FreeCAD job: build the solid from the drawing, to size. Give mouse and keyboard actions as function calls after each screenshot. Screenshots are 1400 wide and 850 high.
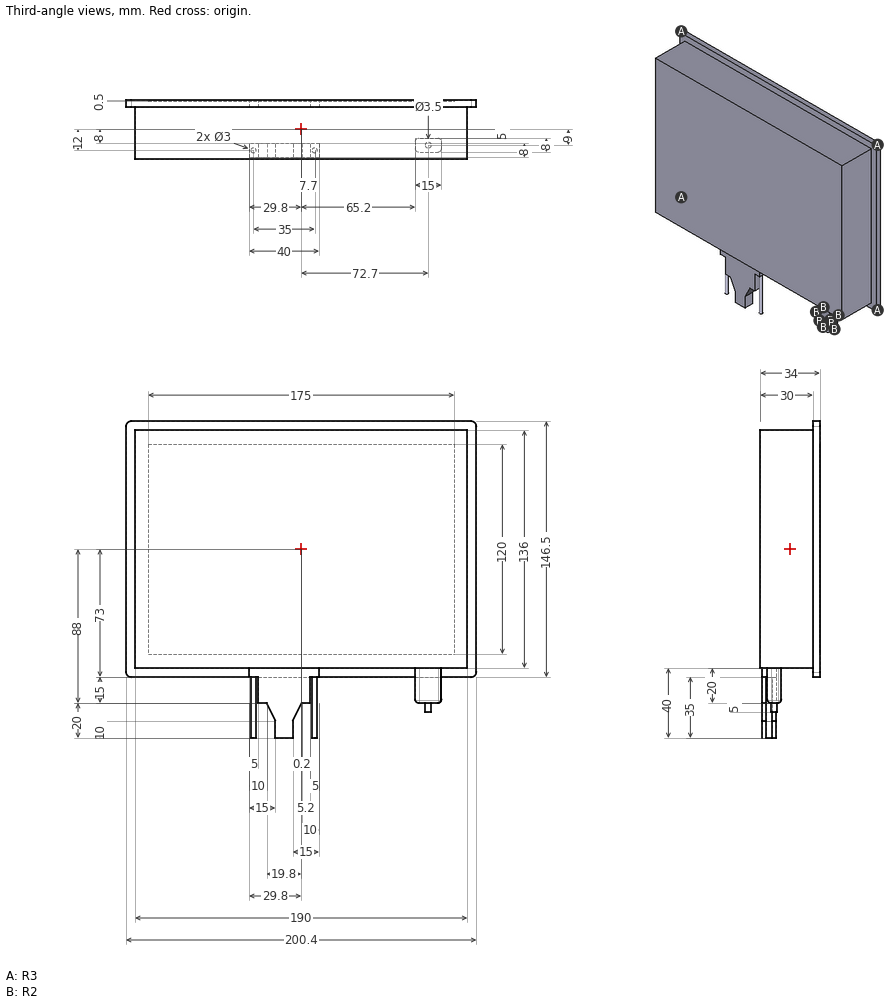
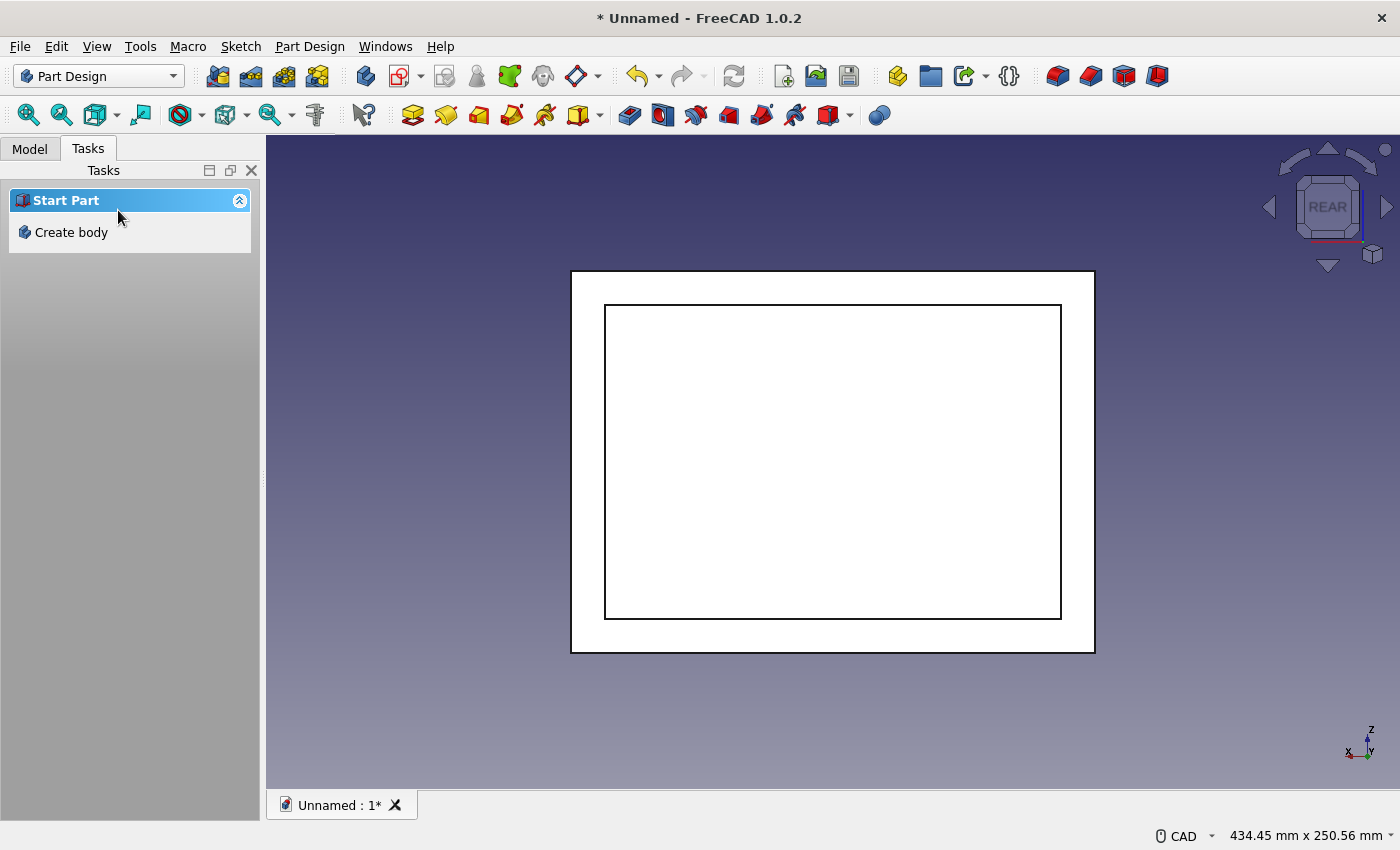
key(0)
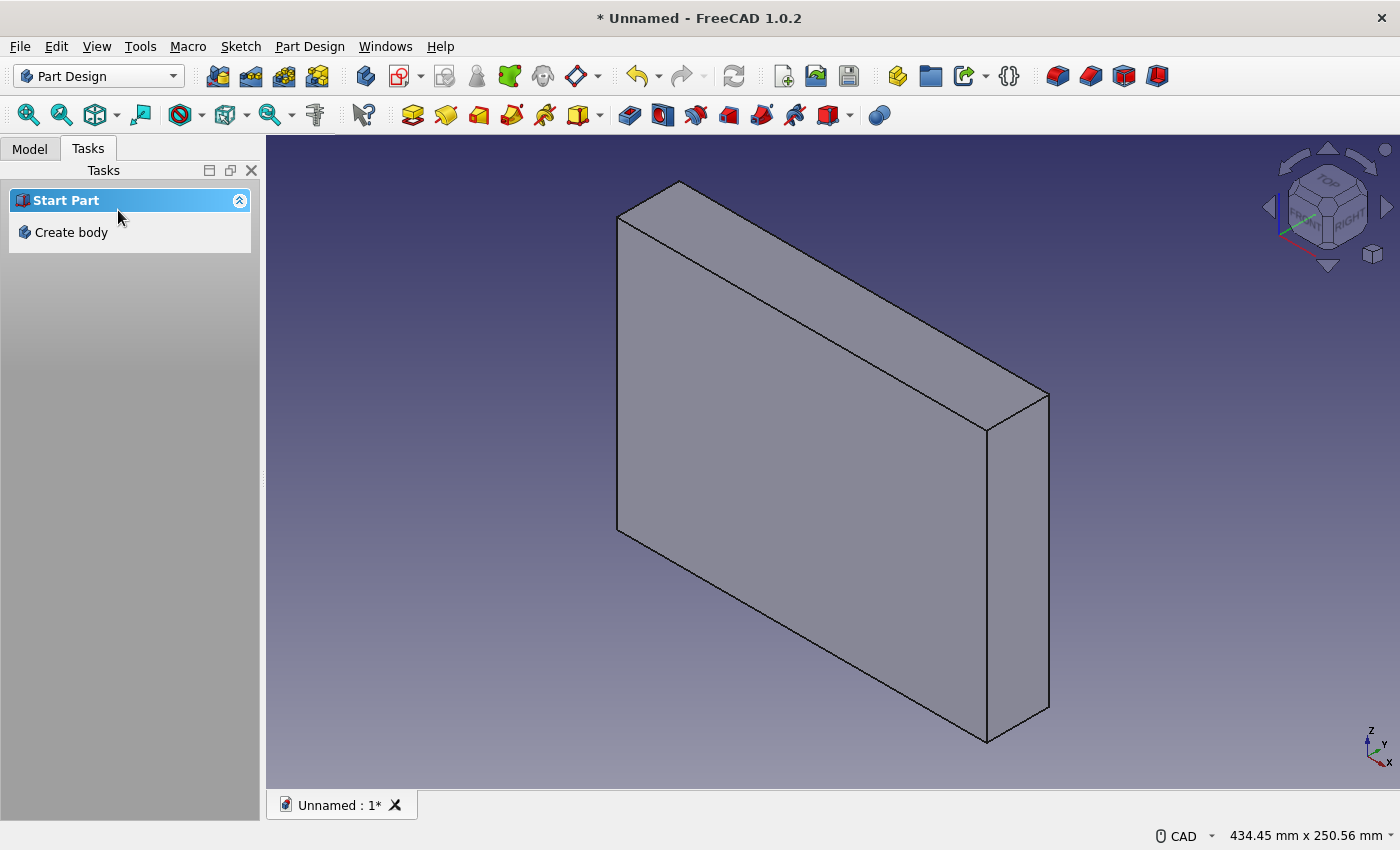
click(802, 479)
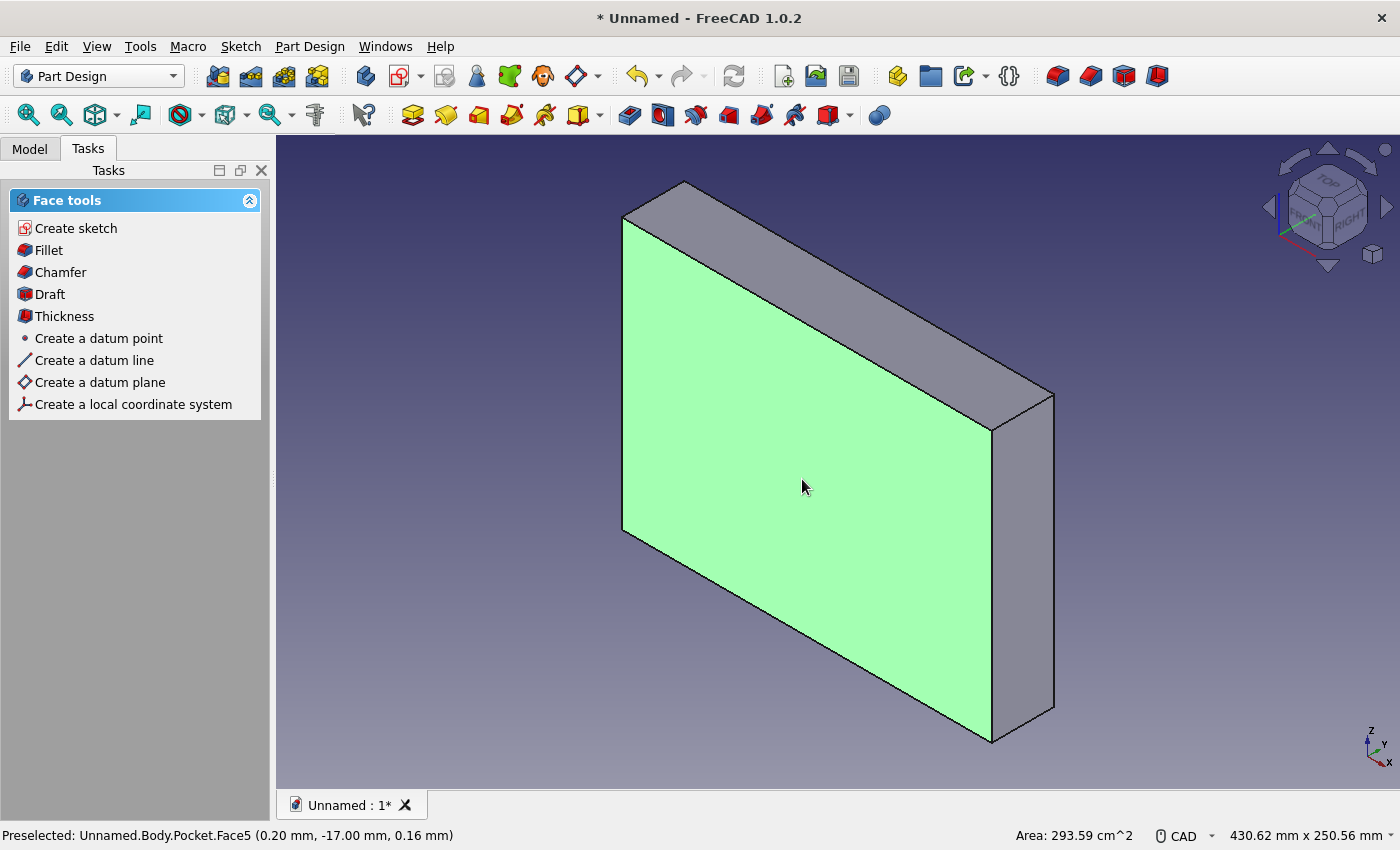
click(398, 76)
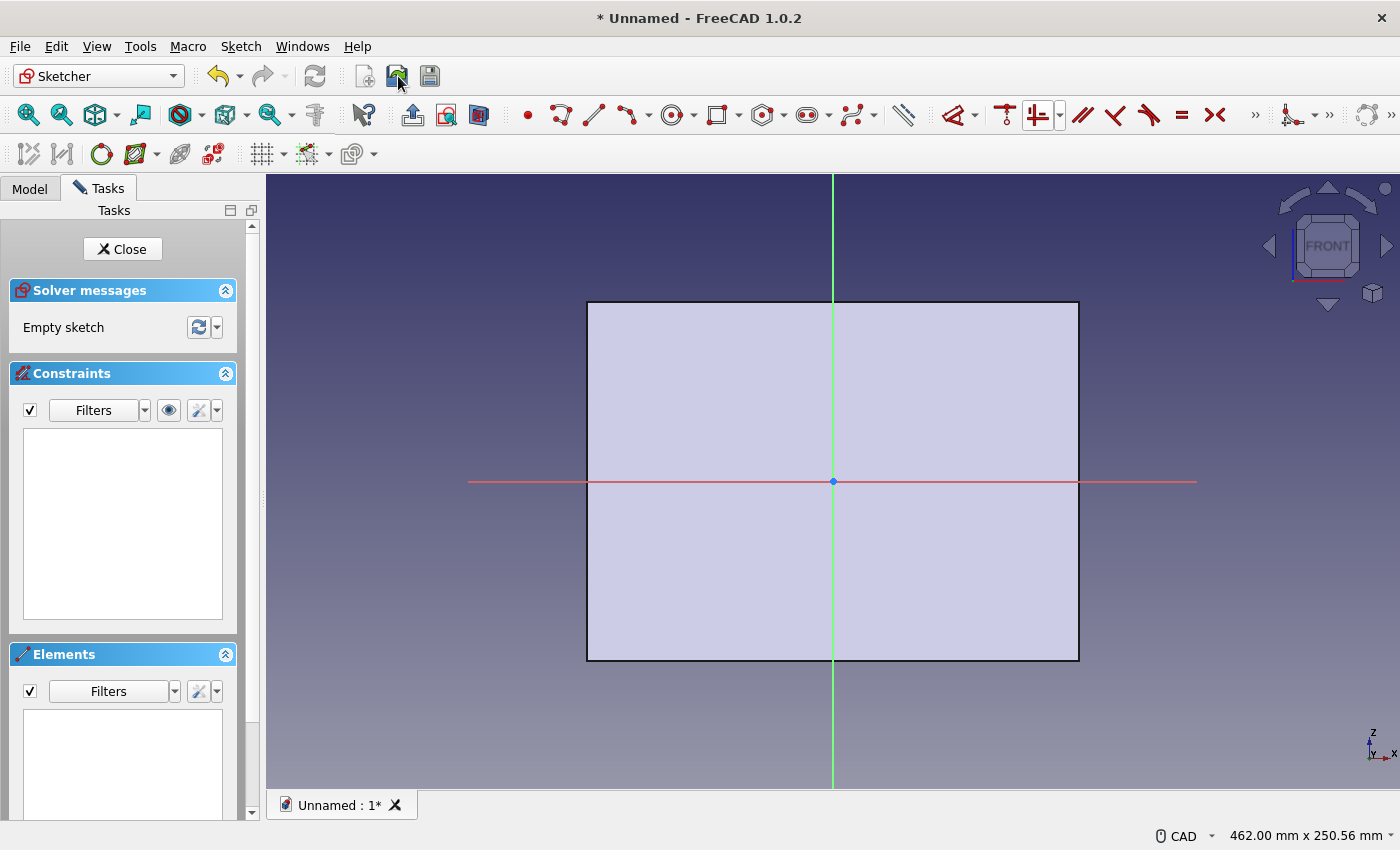
key(g)
key(v)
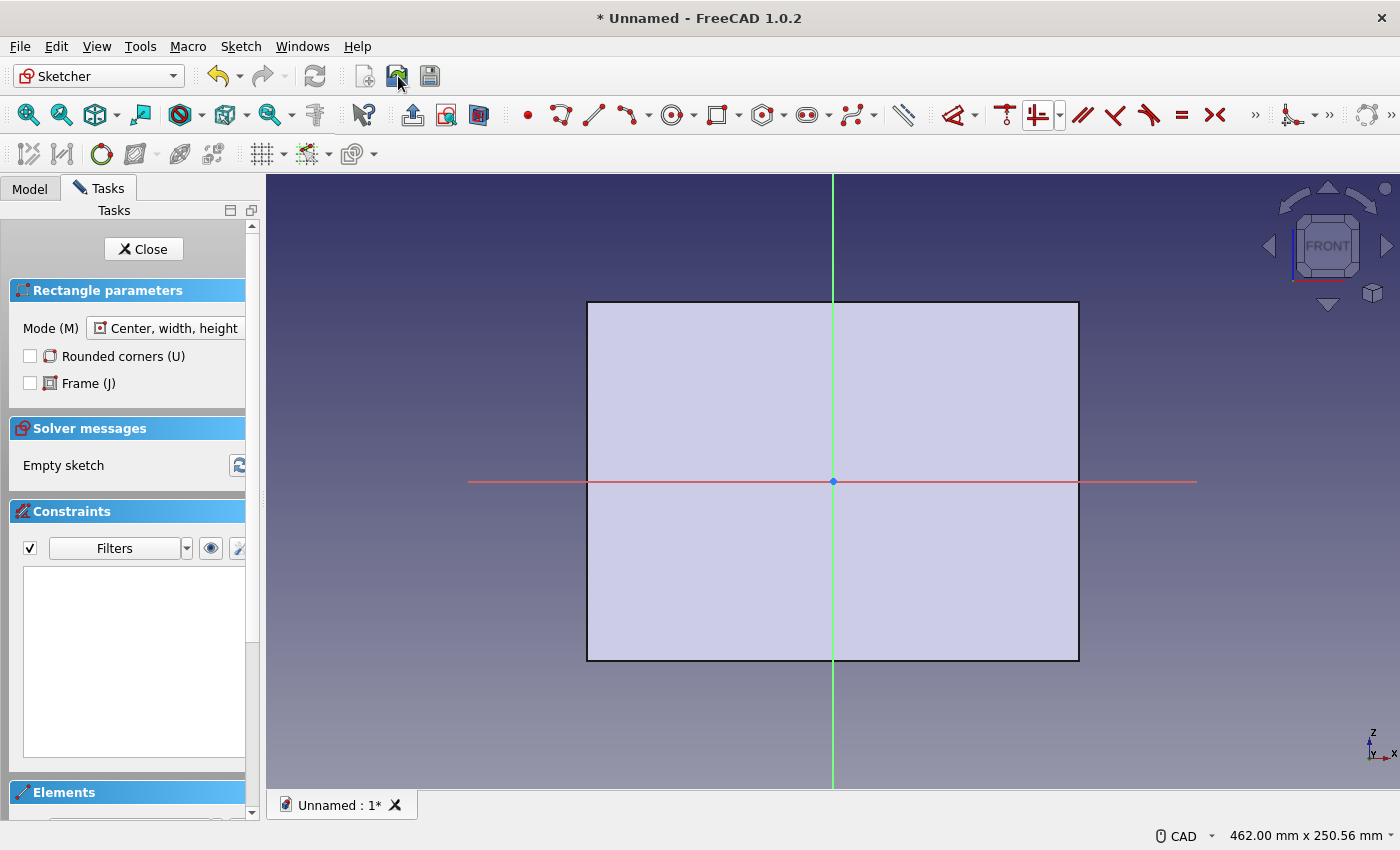
click(833, 482)
move(1079, 302)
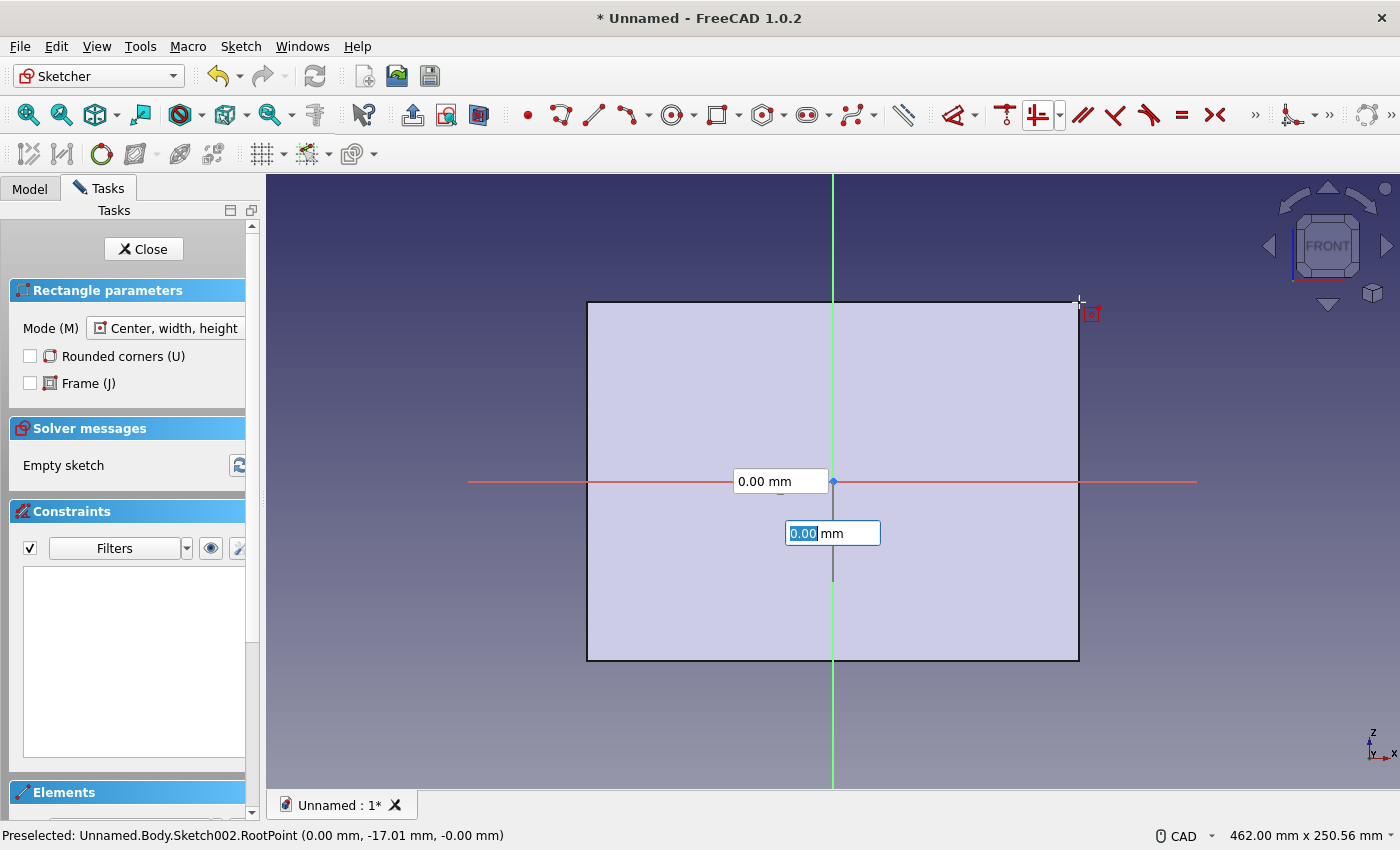
text(200.4)
key(Tab)
text(146.5)
key(Return)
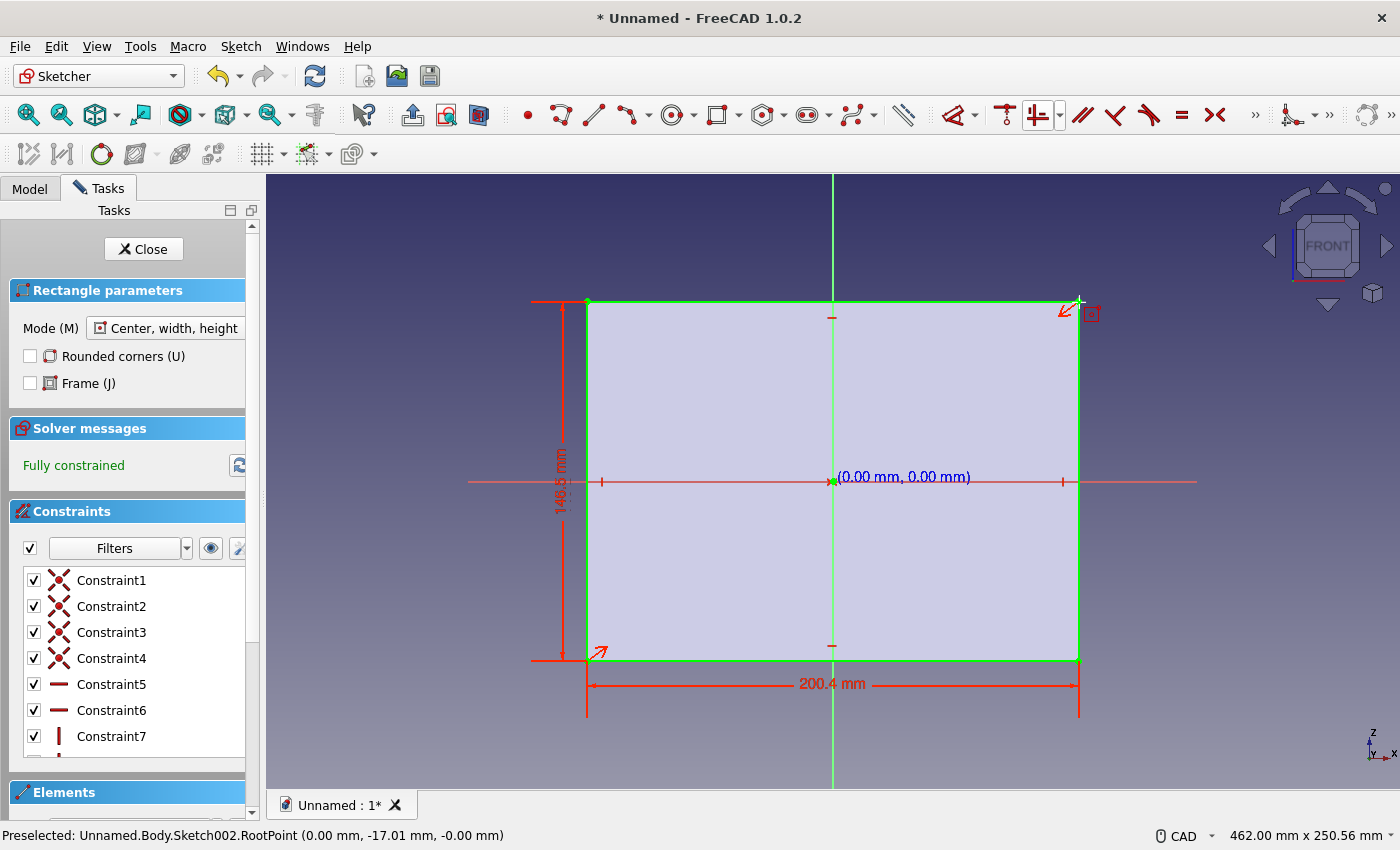
click(833, 482)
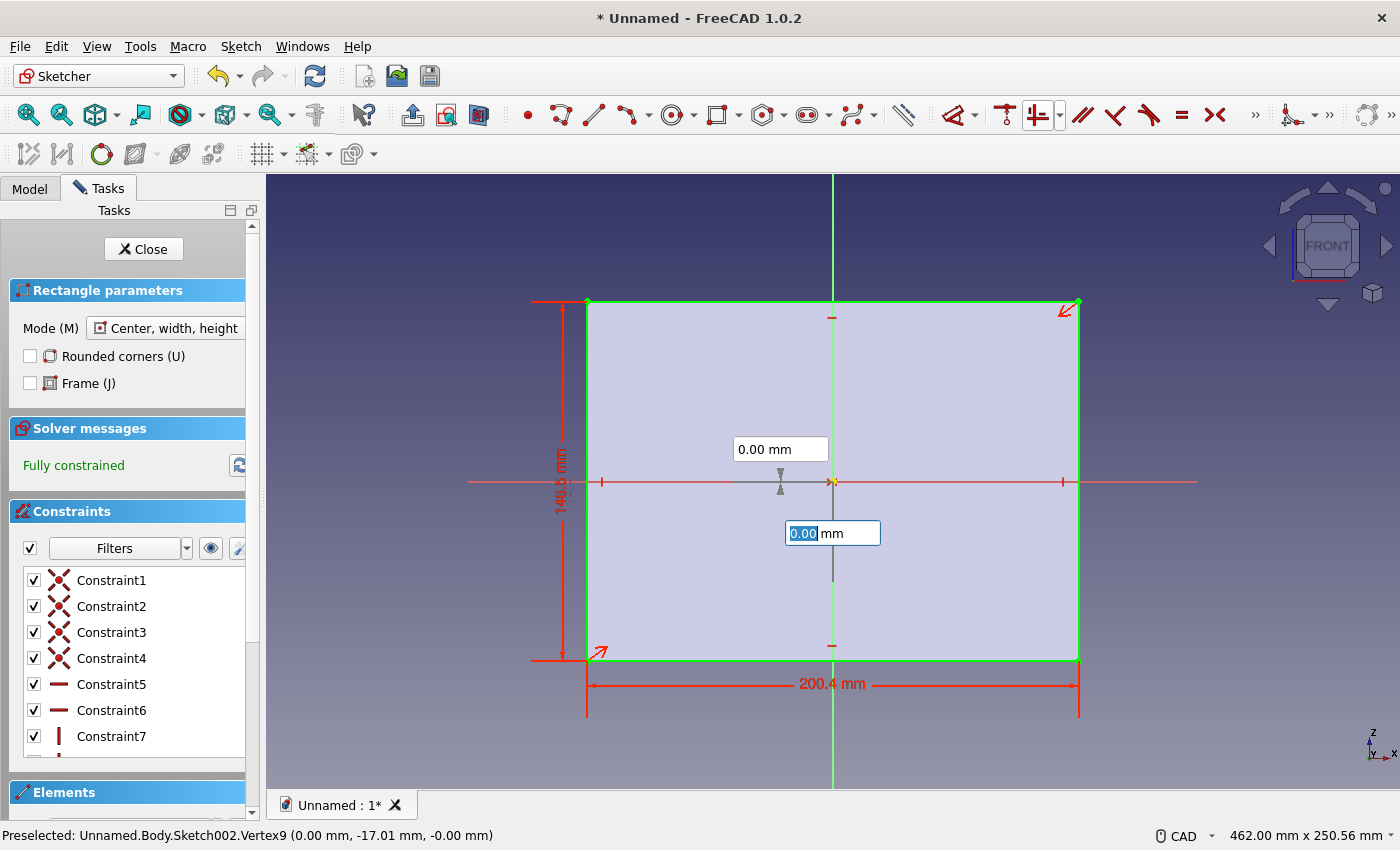
scroll(1066, 315, up, 2)
move(1066, 314)